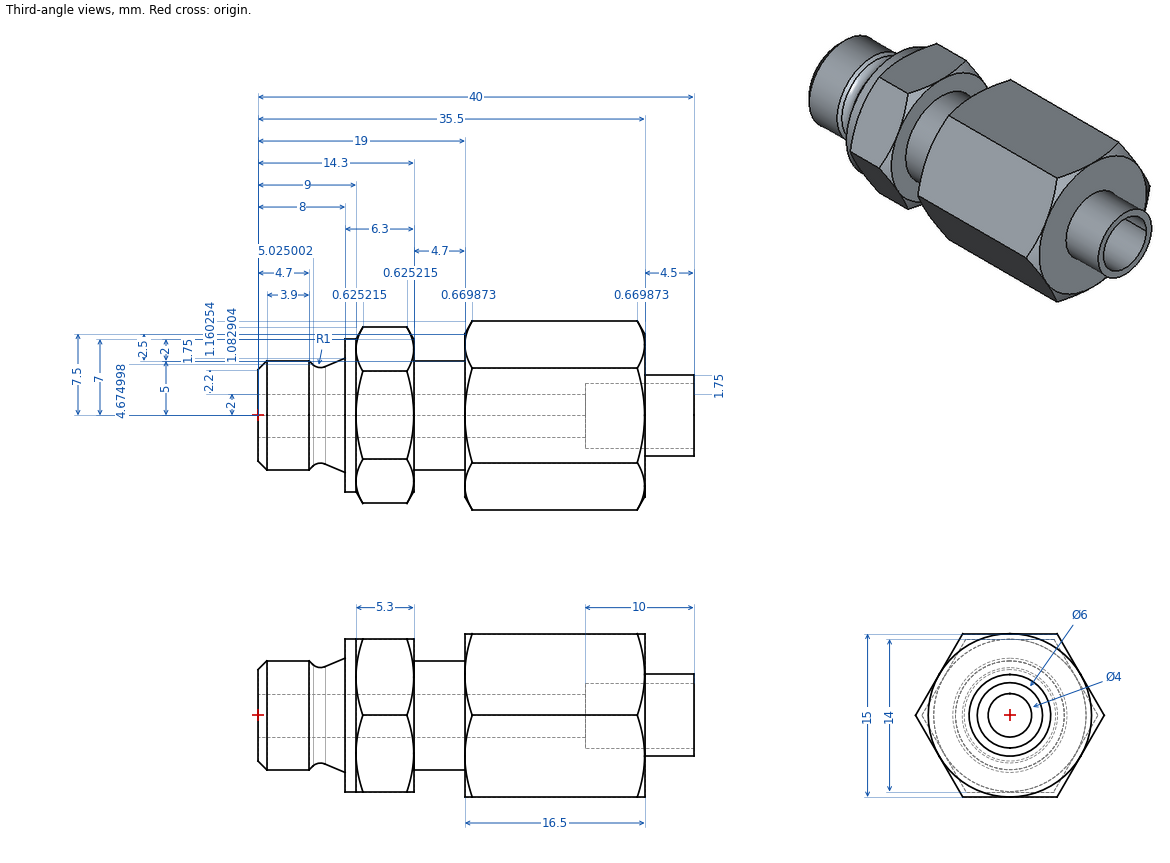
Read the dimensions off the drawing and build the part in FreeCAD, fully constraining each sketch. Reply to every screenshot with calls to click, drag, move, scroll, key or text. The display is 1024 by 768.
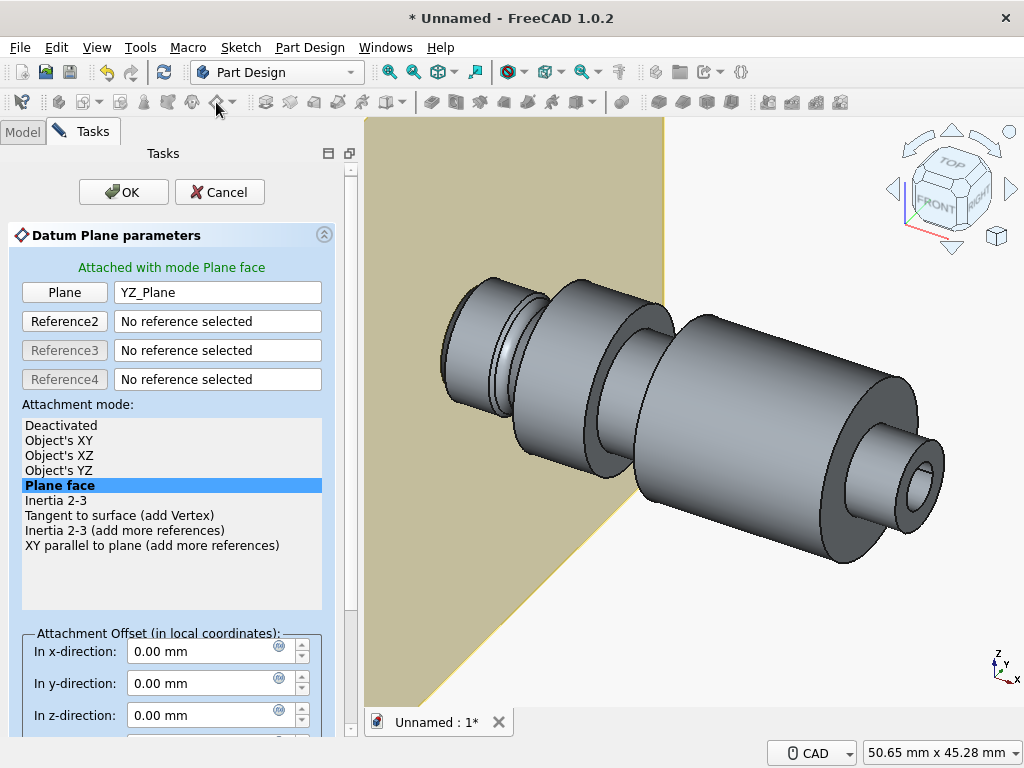
triple_click(210, 715)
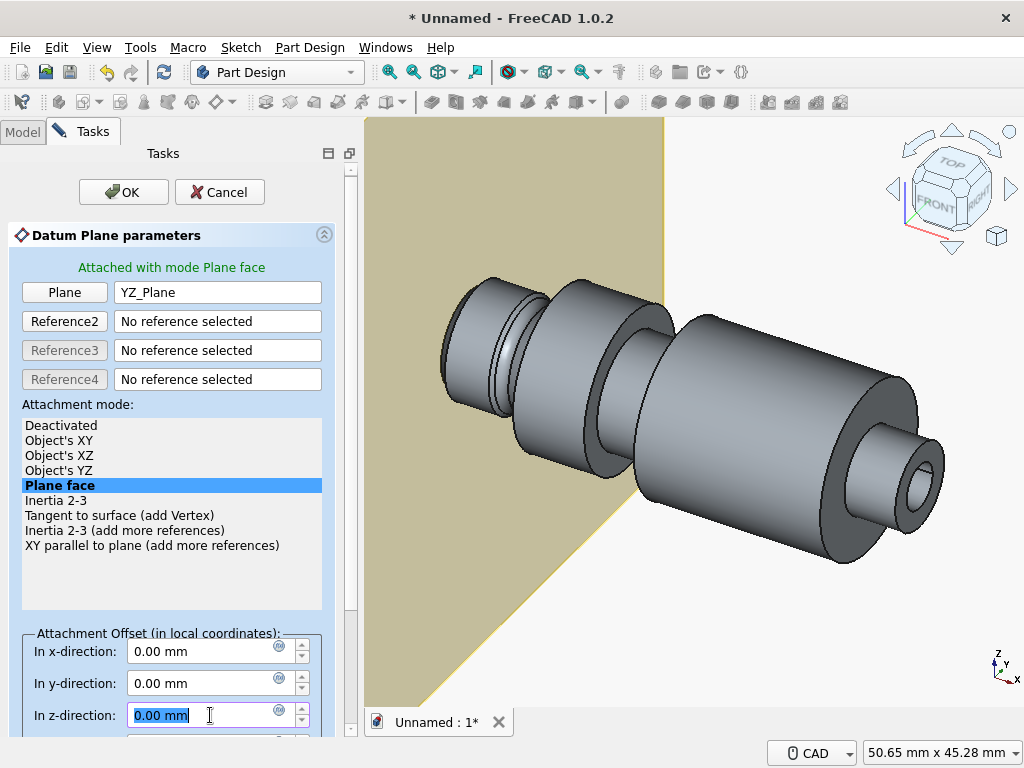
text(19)
key(Tab)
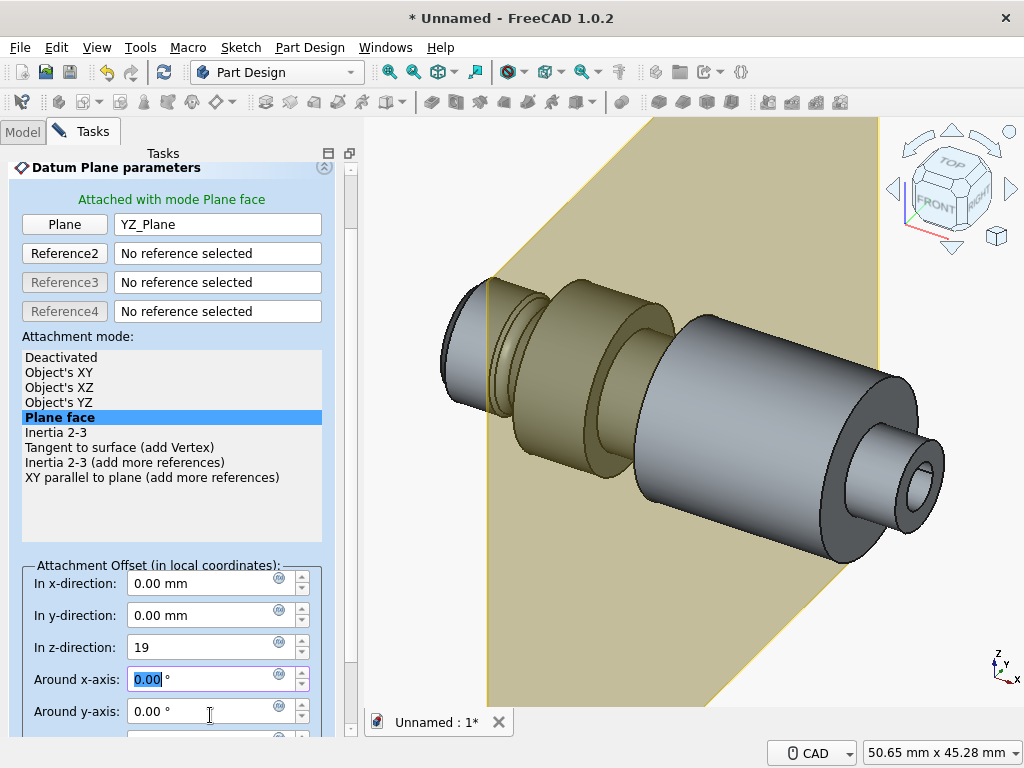
scroll(351, 450, up, 2)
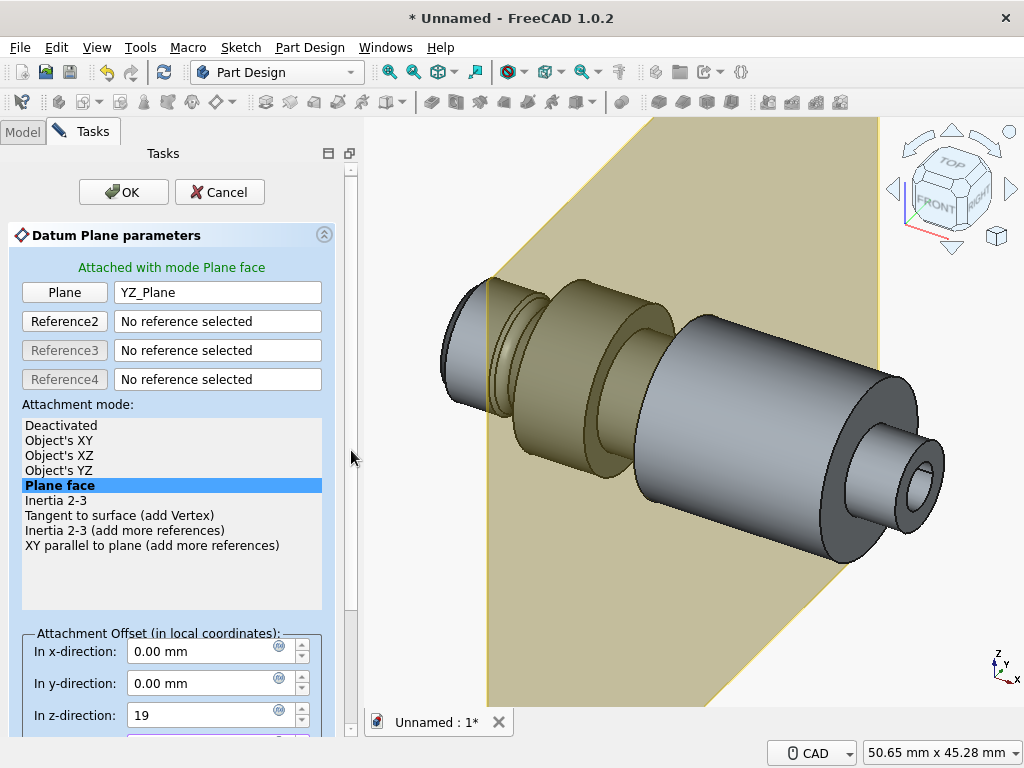
click(124, 192)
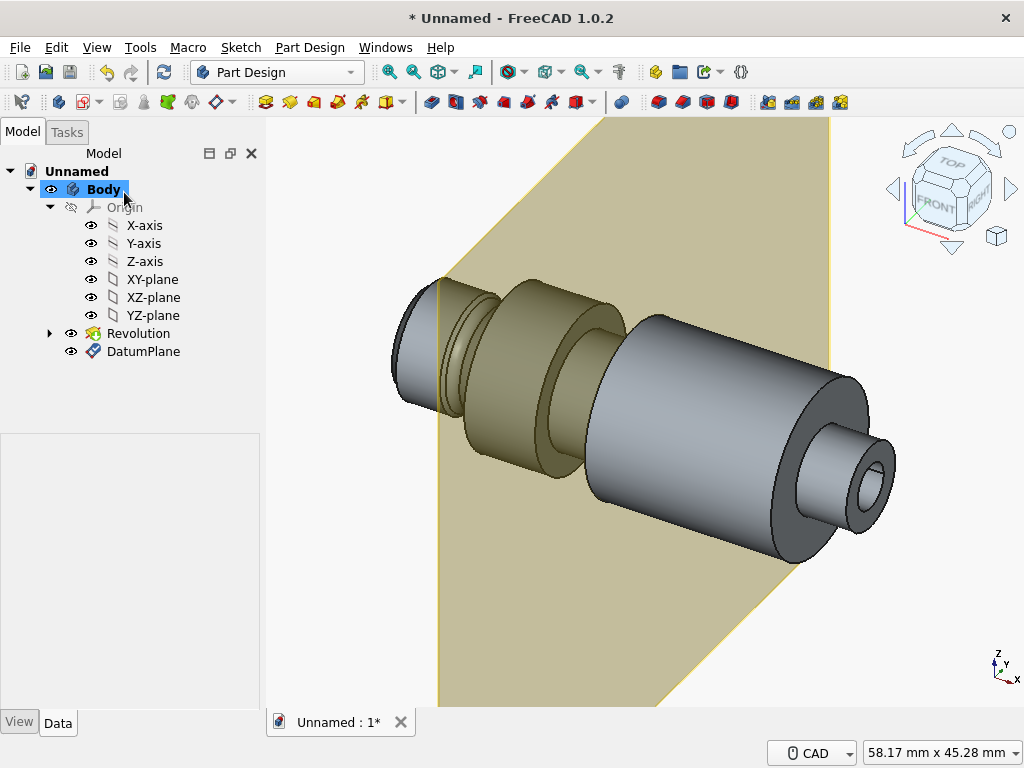
click(116, 351)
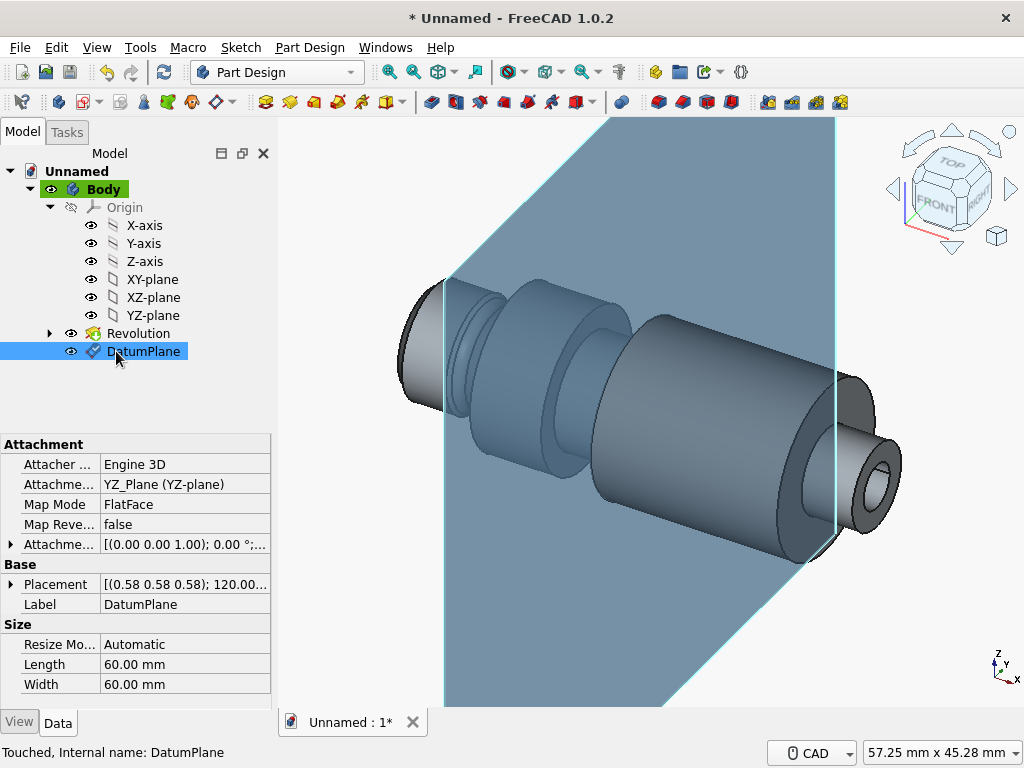
click(84, 102)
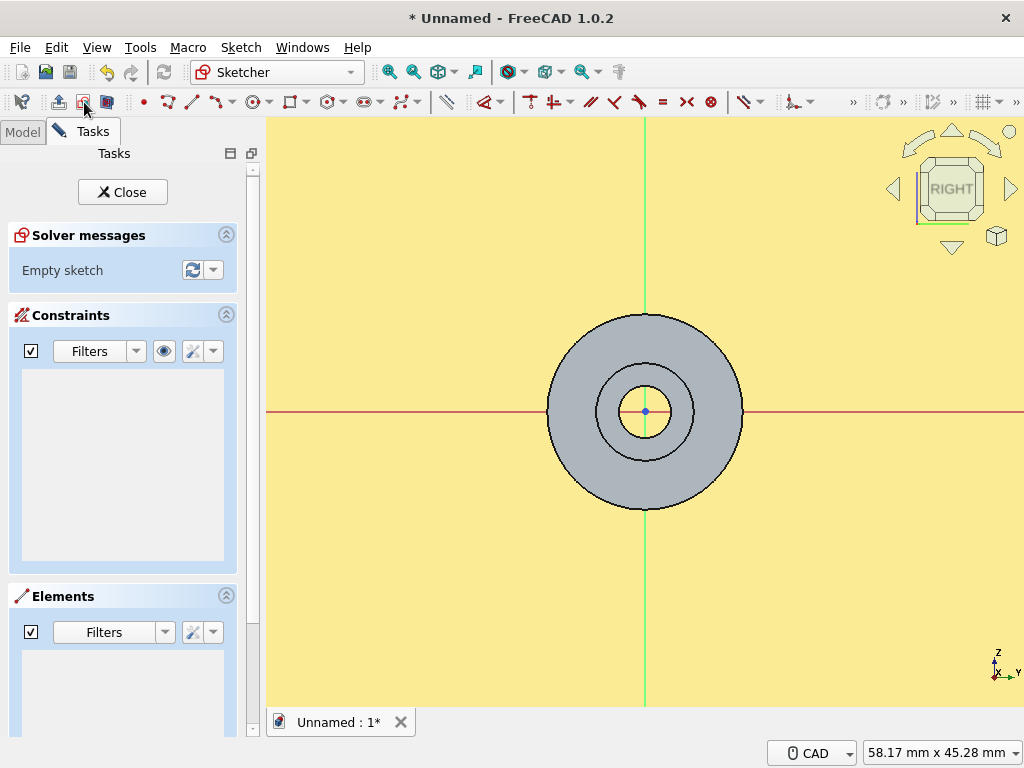
click(108, 102)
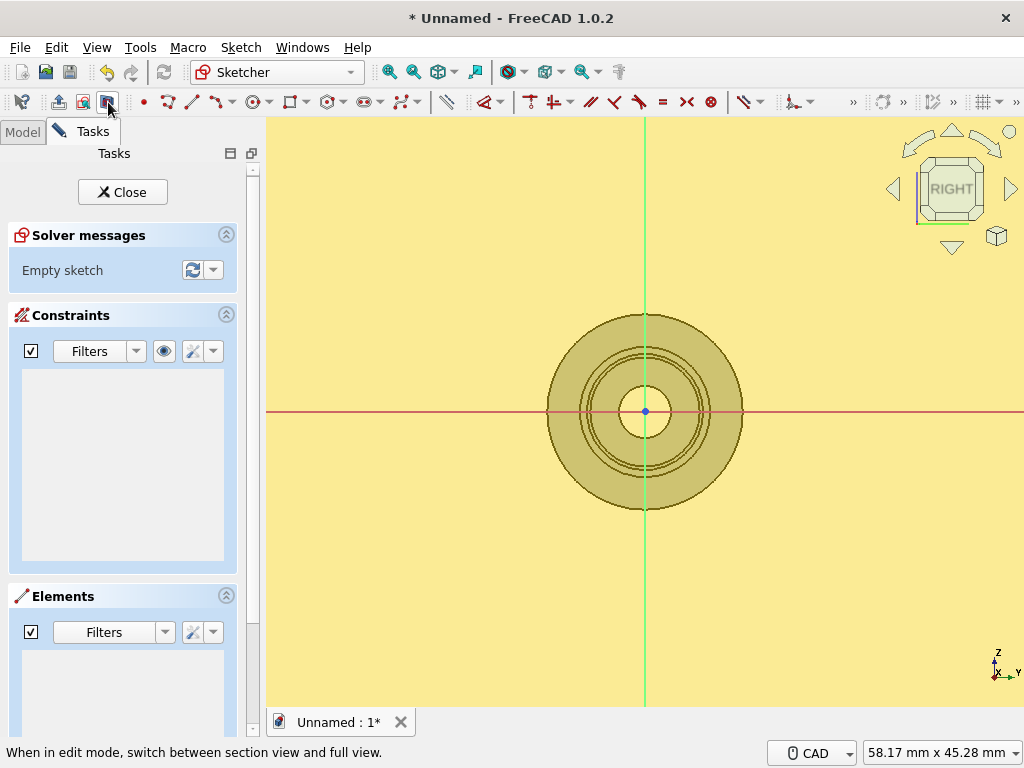
scroll(728, 412, up, 3)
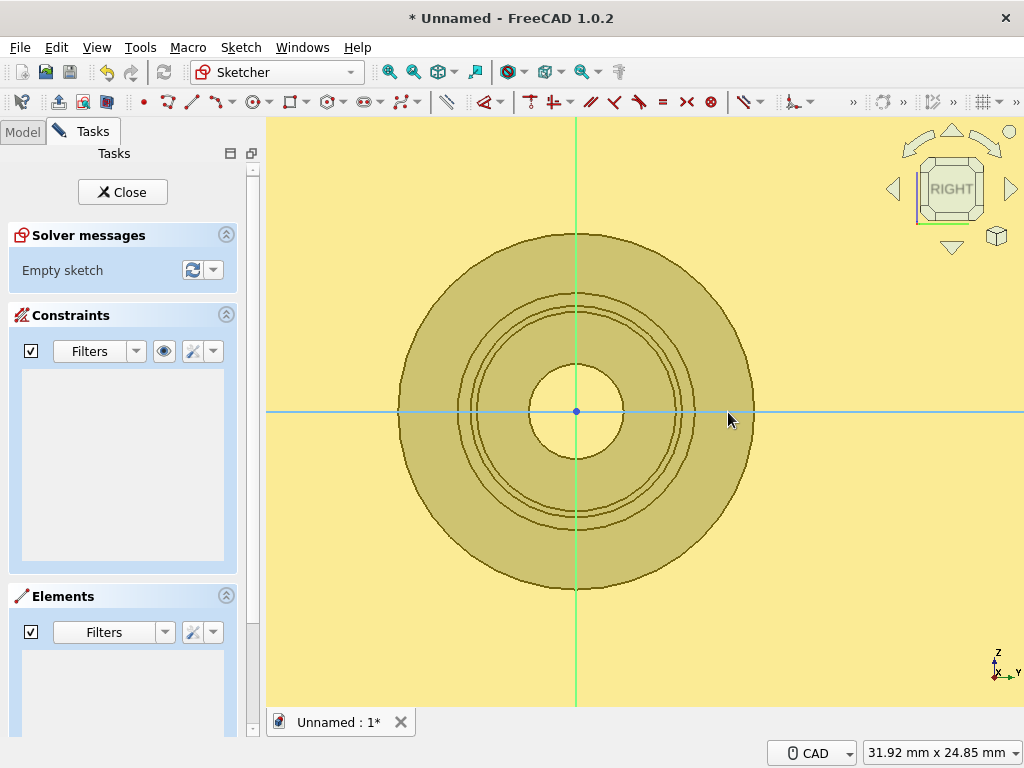
click(328, 102)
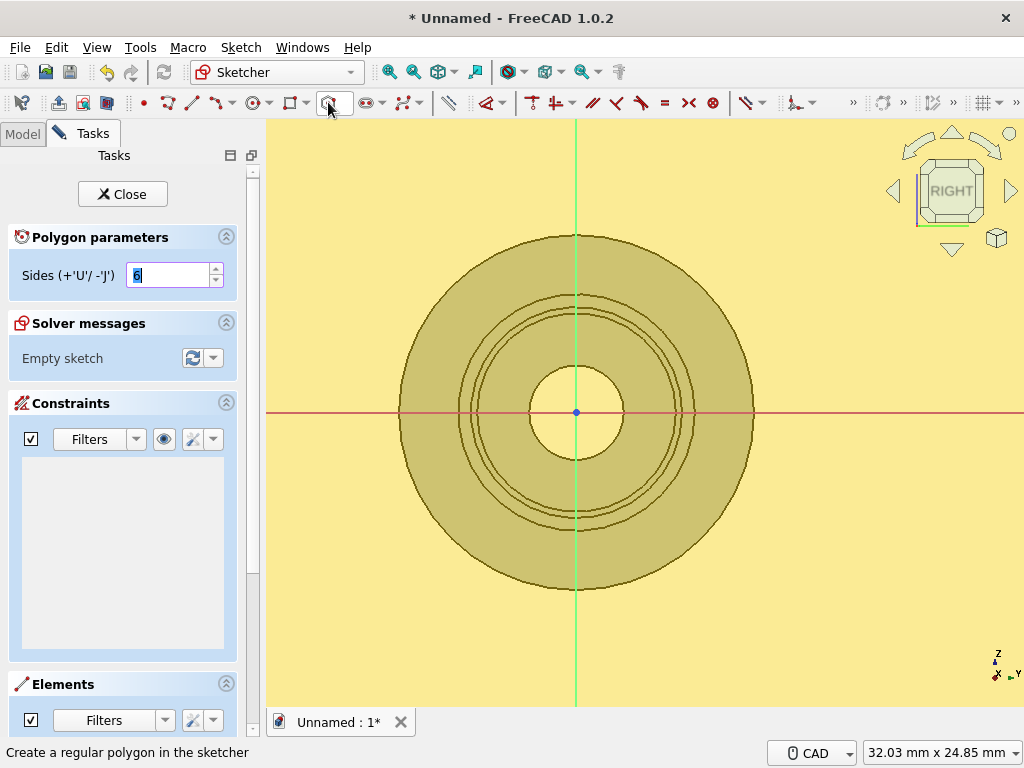
click(576, 413)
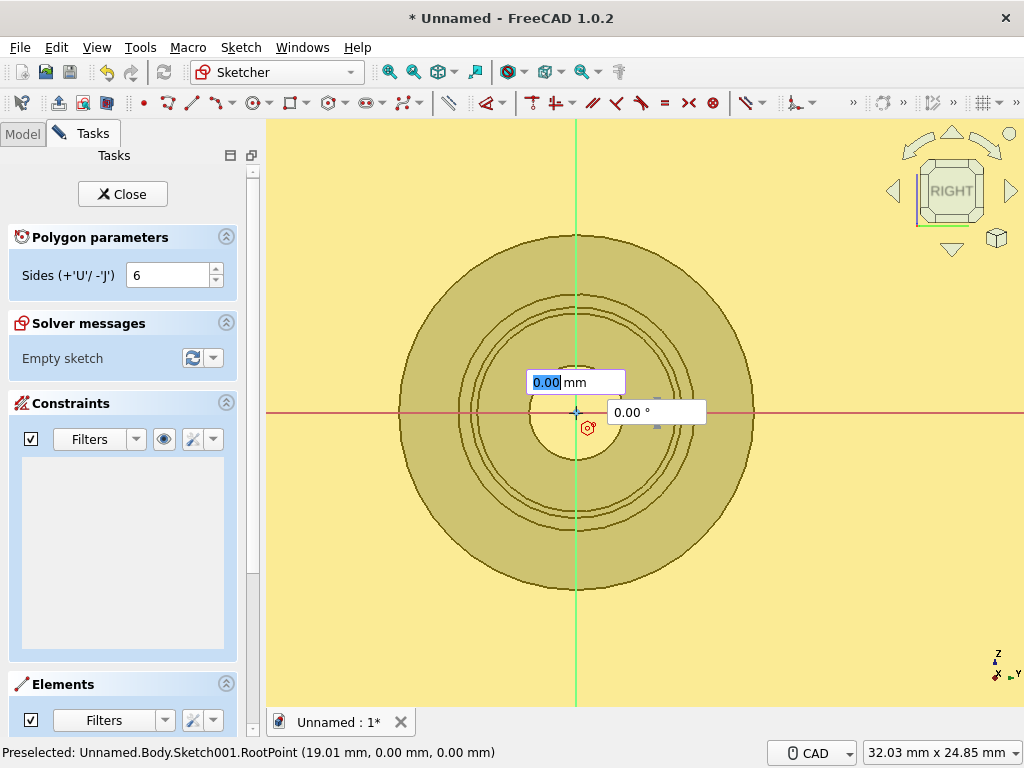
click(781, 413)
right_click(781, 413)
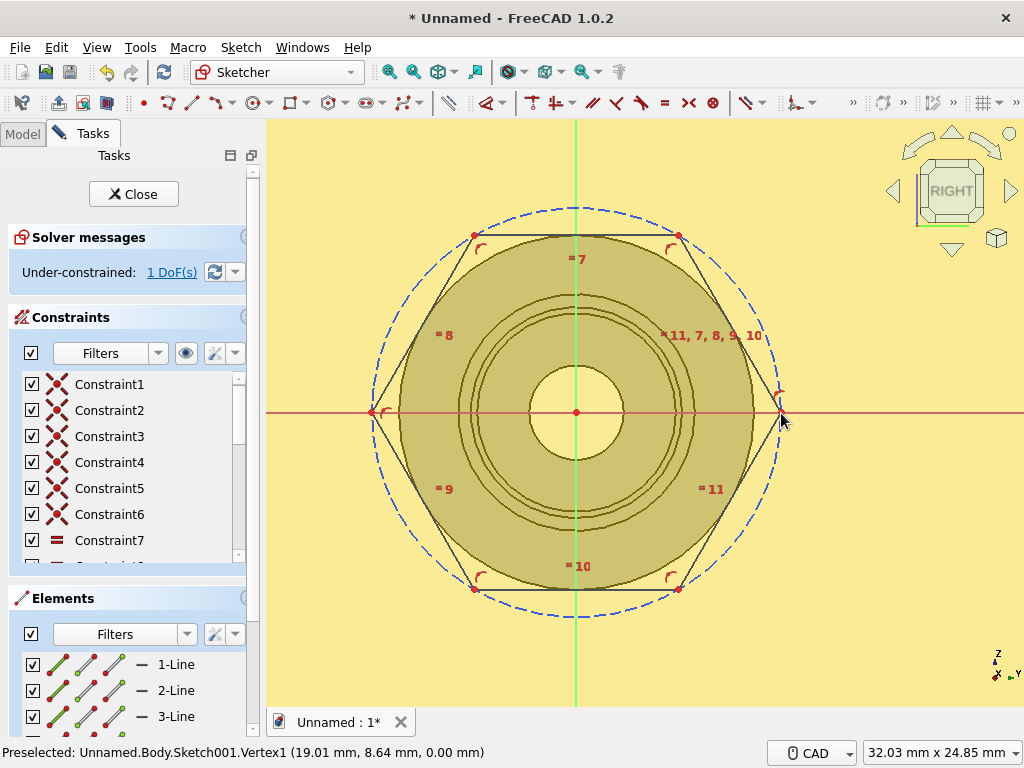
click(254, 104)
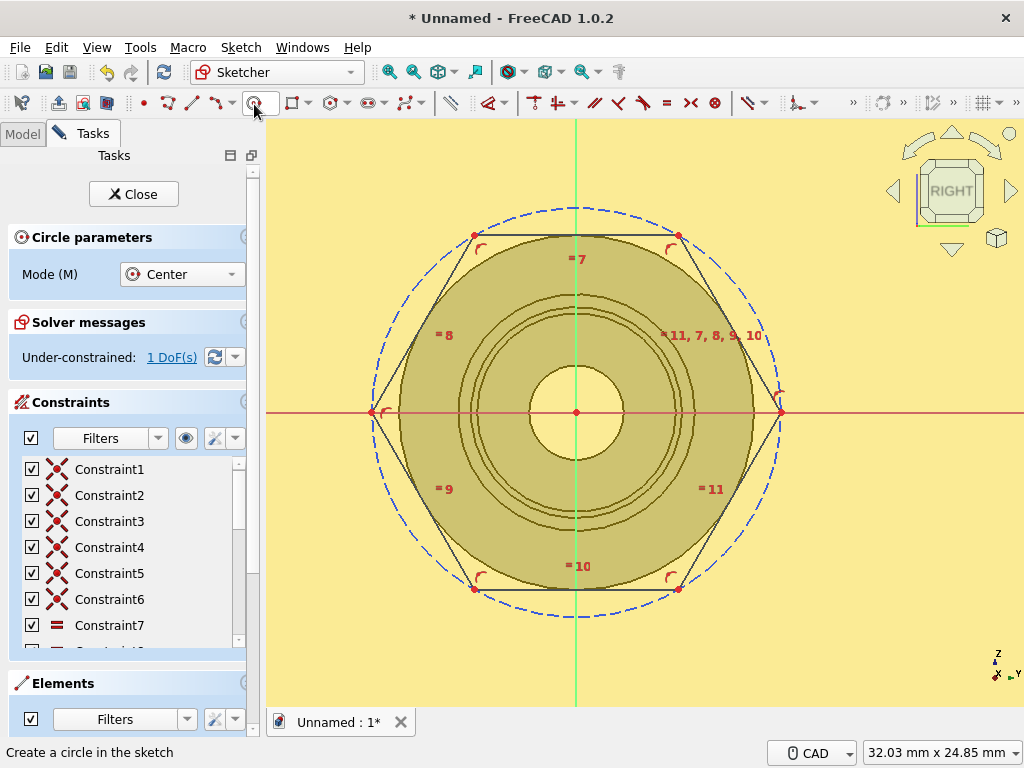
click(576, 413)
click(610, 379)
key(Escape)